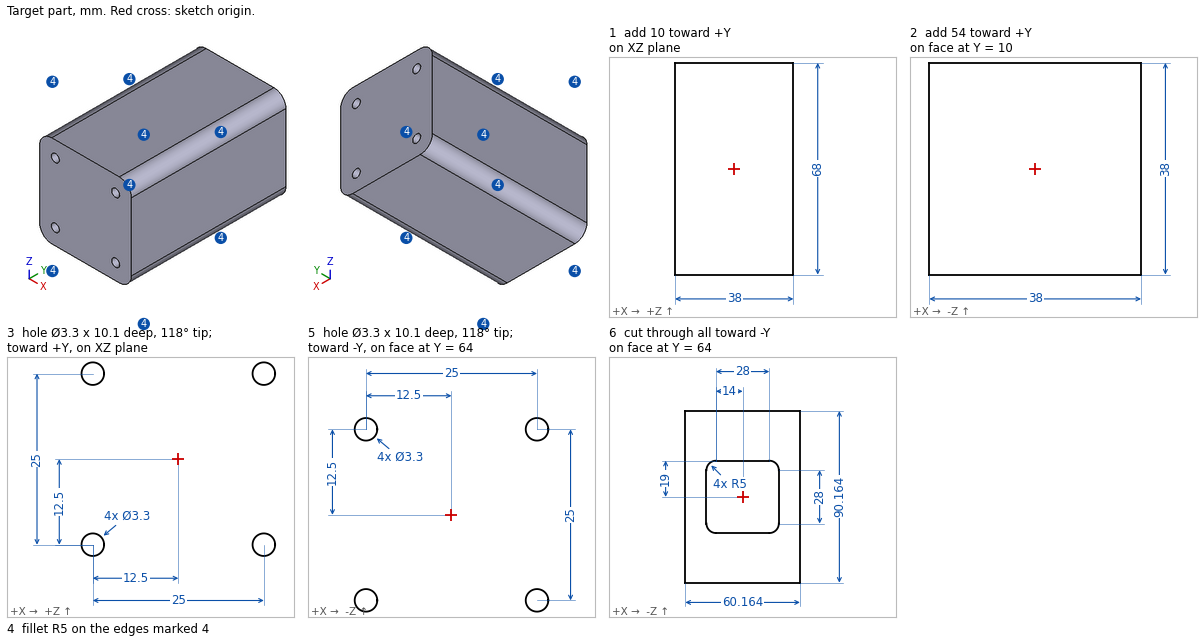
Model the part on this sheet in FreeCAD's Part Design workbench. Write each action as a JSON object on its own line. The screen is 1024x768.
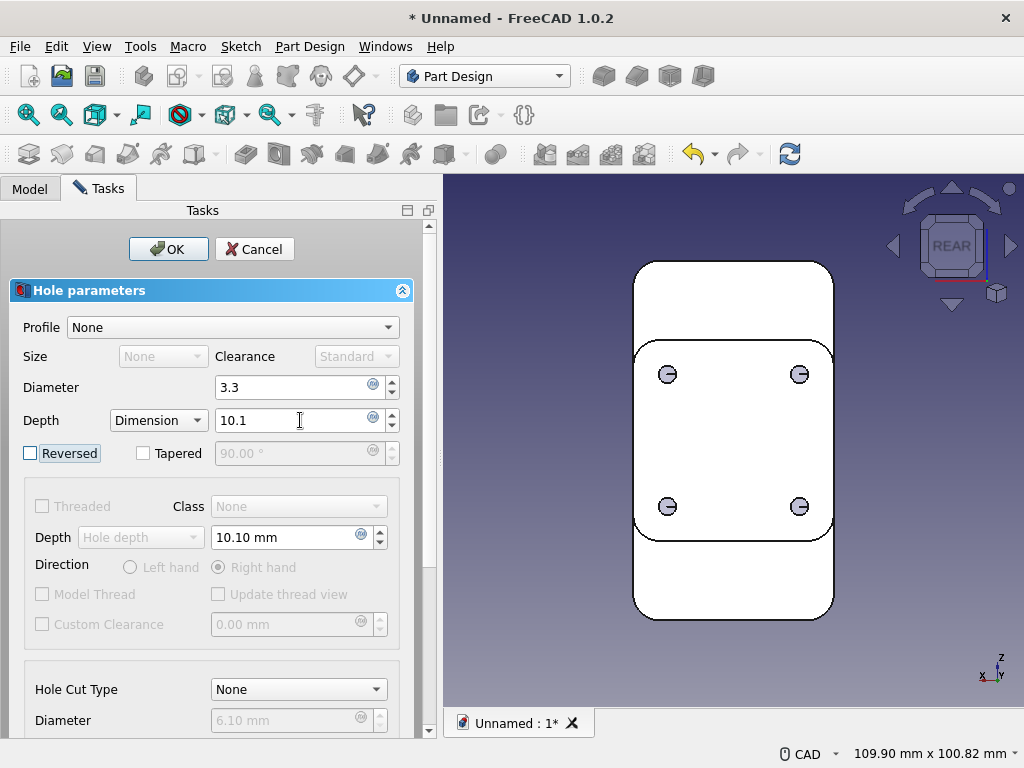
{"action": "left_click", "coordinate": [169, 249]}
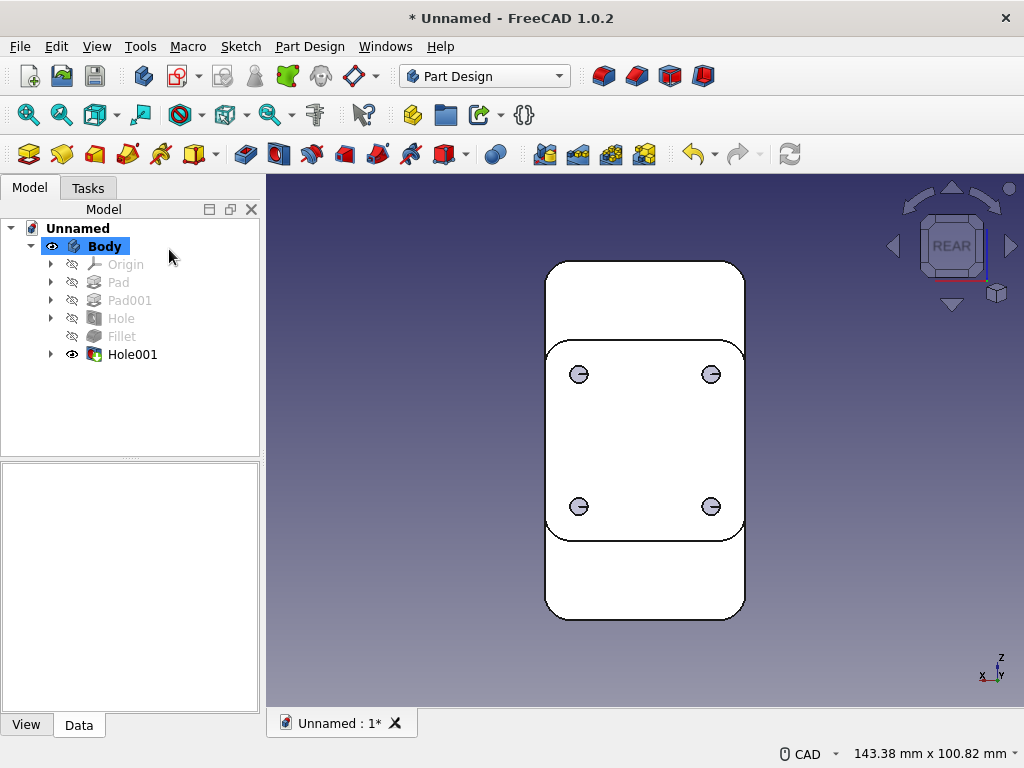
{"action": "left_click", "coordinate": [645, 440]}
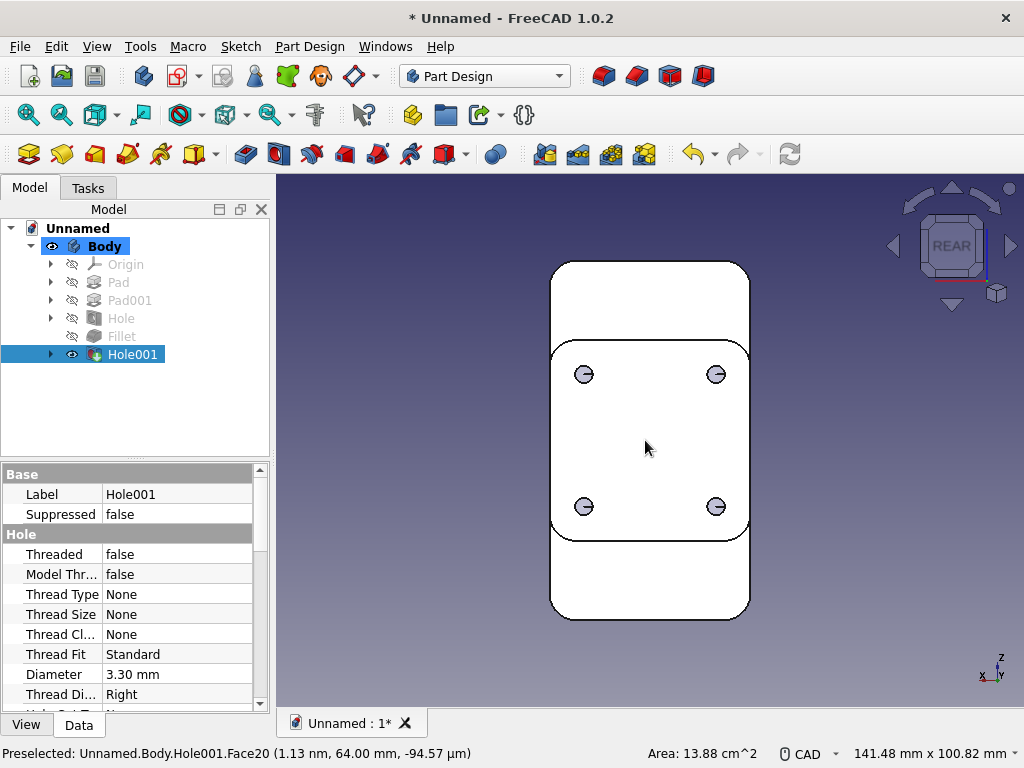
{"action": "left_click", "coordinate": [176, 76]}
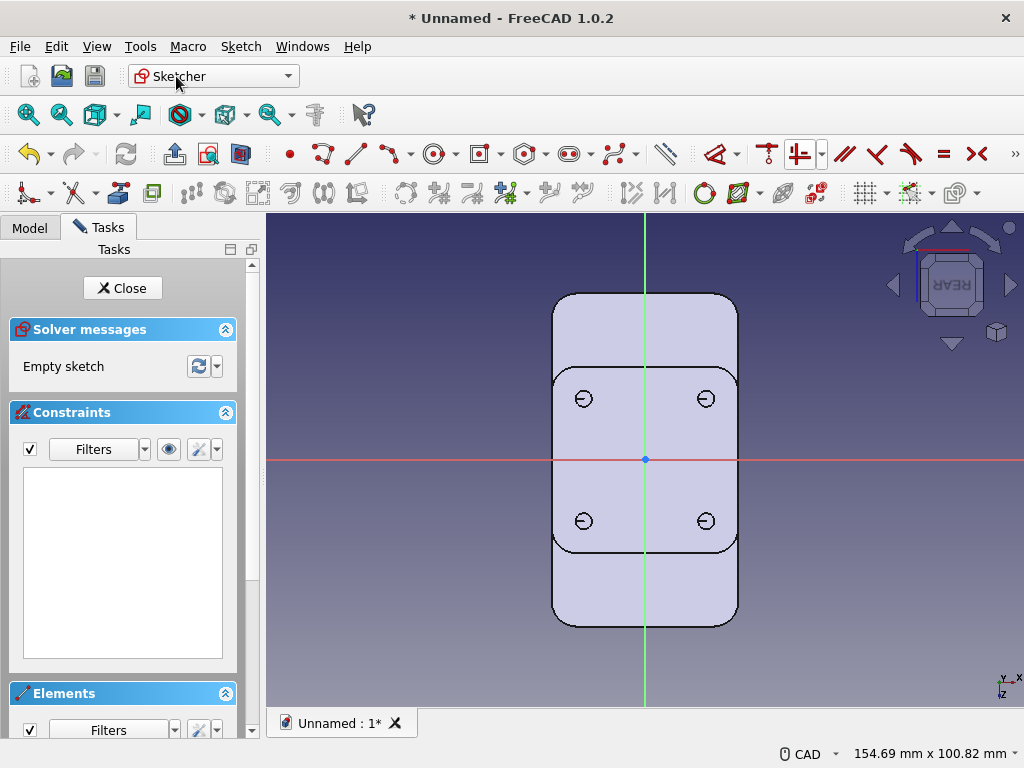
{"action": "scroll", "coordinate": [437, 460], "scroll_direction": "down", "scroll_amount": 2}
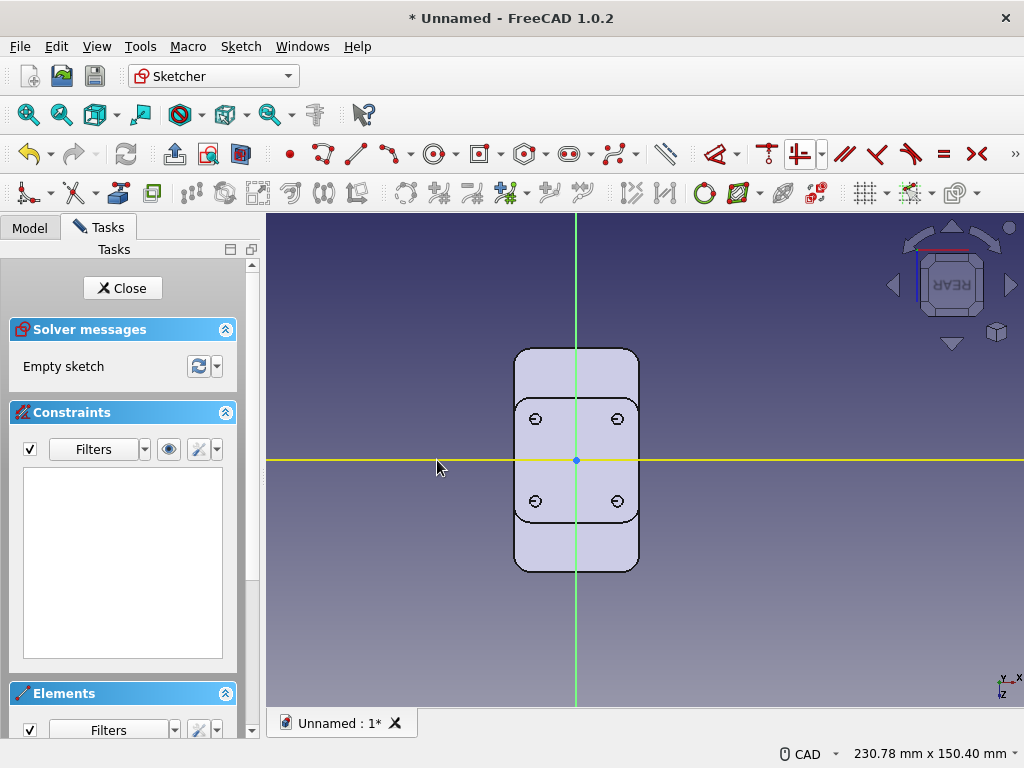
{"action": "key", "text": "g v"}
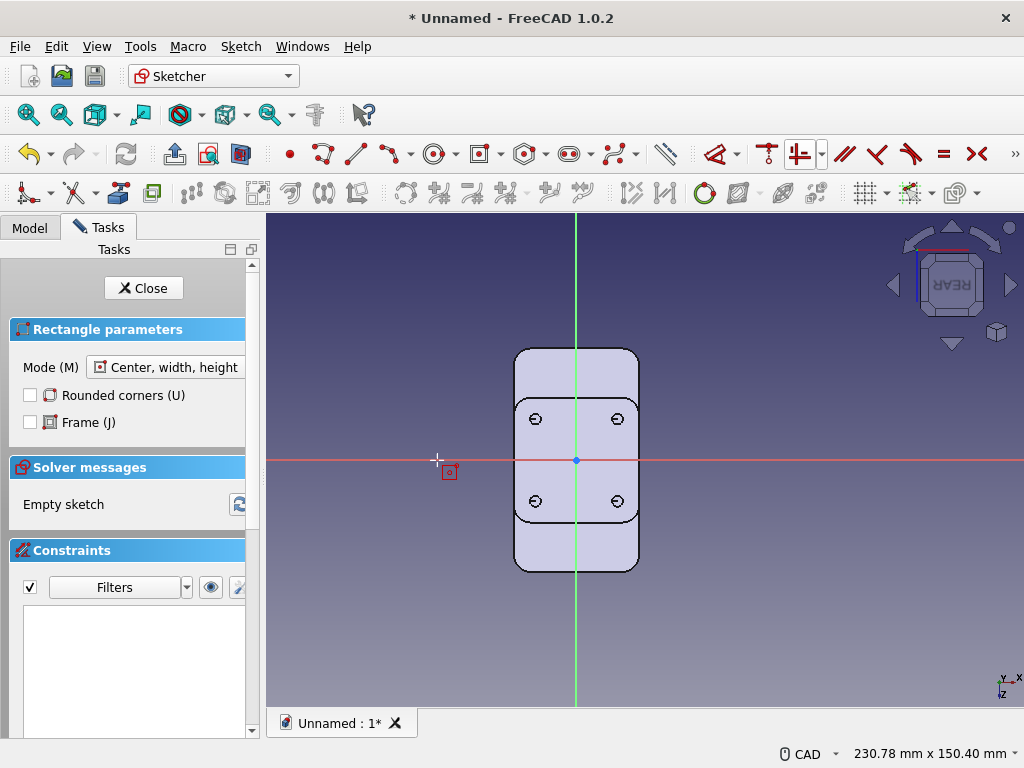
{"action": "left_click", "coordinate": [577, 460]}
{"action": "left_click", "coordinate": [675, 312]}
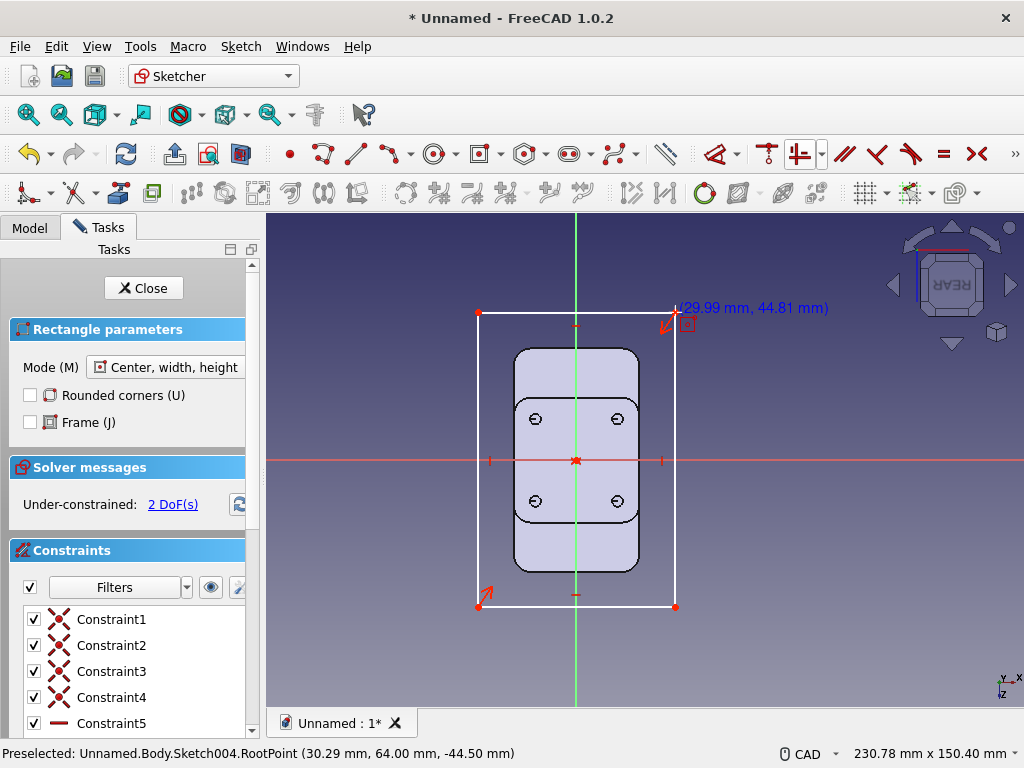
{"action": "left_click", "coordinate": [356, 154]}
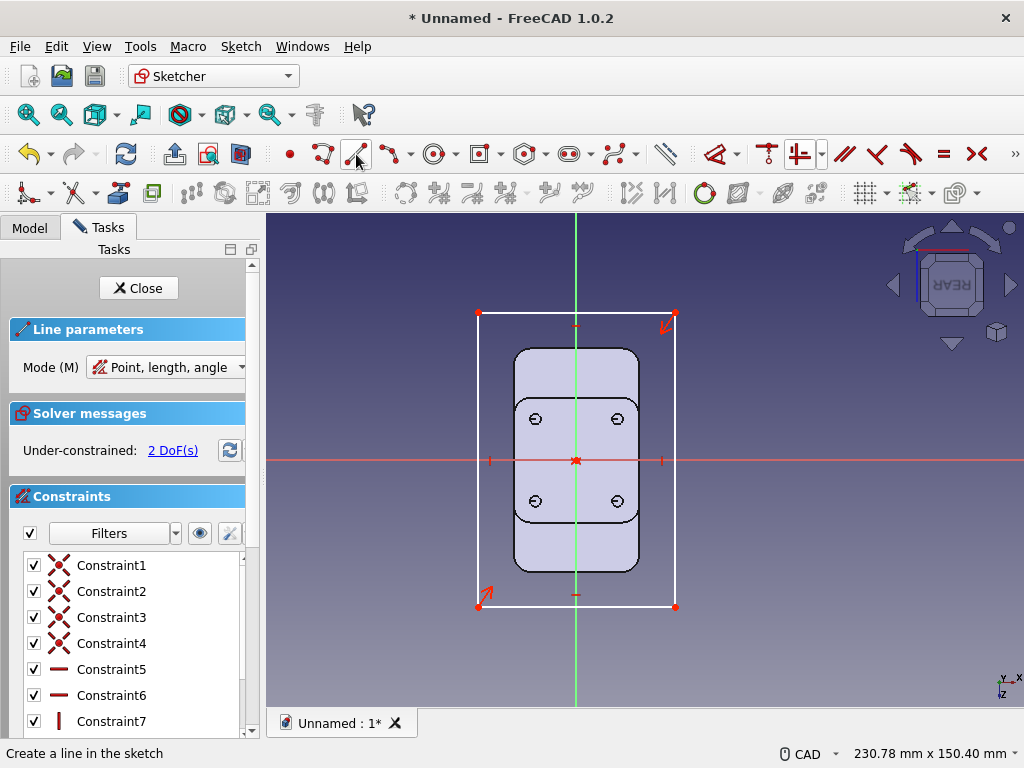
{"action": "left_click", "coordinate": [531, 398]}
{"action": "left_click", "coordinate": [622, 398]}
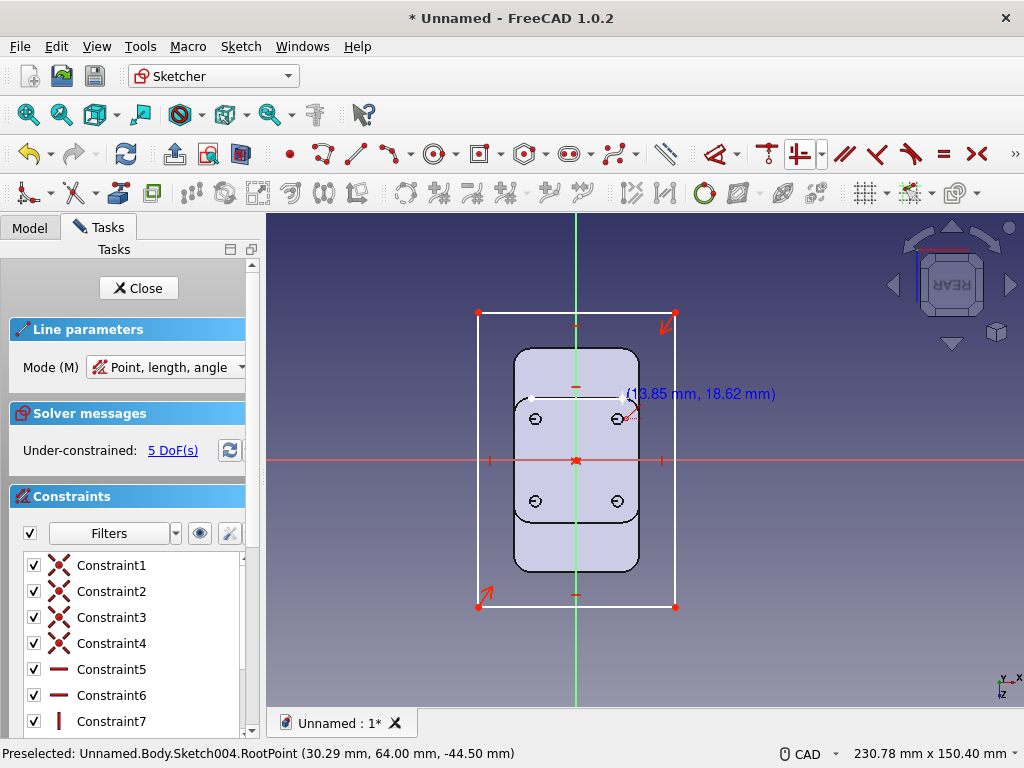
{"action": "left_click", "coordinate": [639, 414]}
{"action": "left_click", "coordinate": [639, 506]}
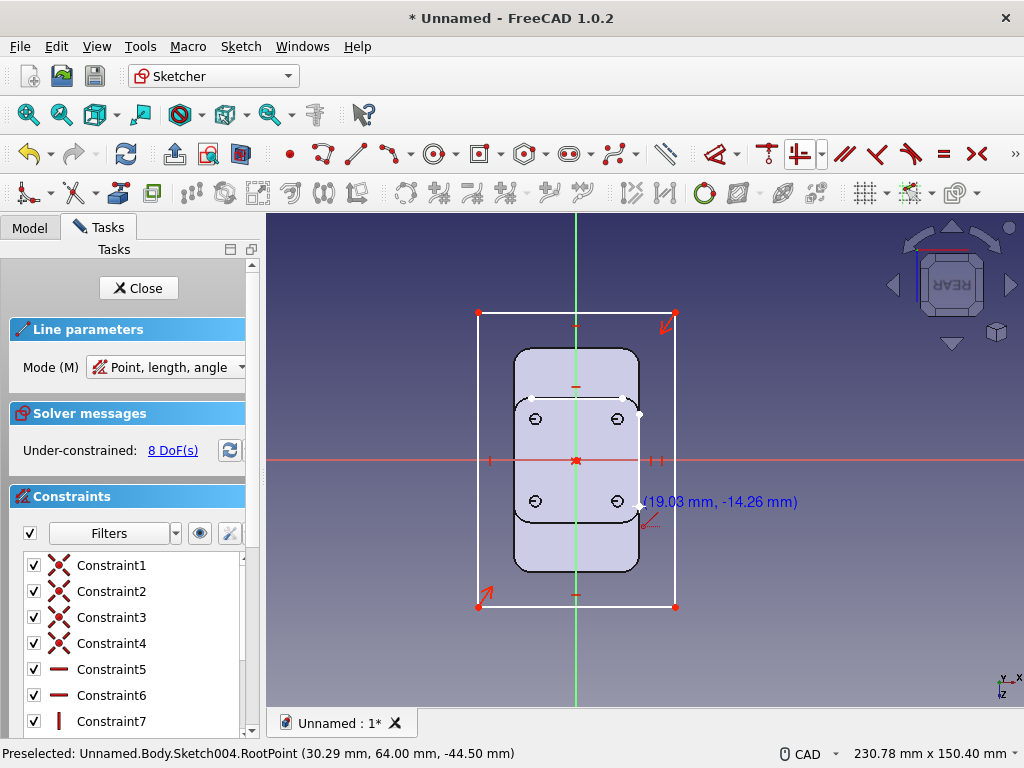
{"action": "left_click", "coordinate": [622, 523]}
{"action": "left_click", "coordinate": [531, 523]}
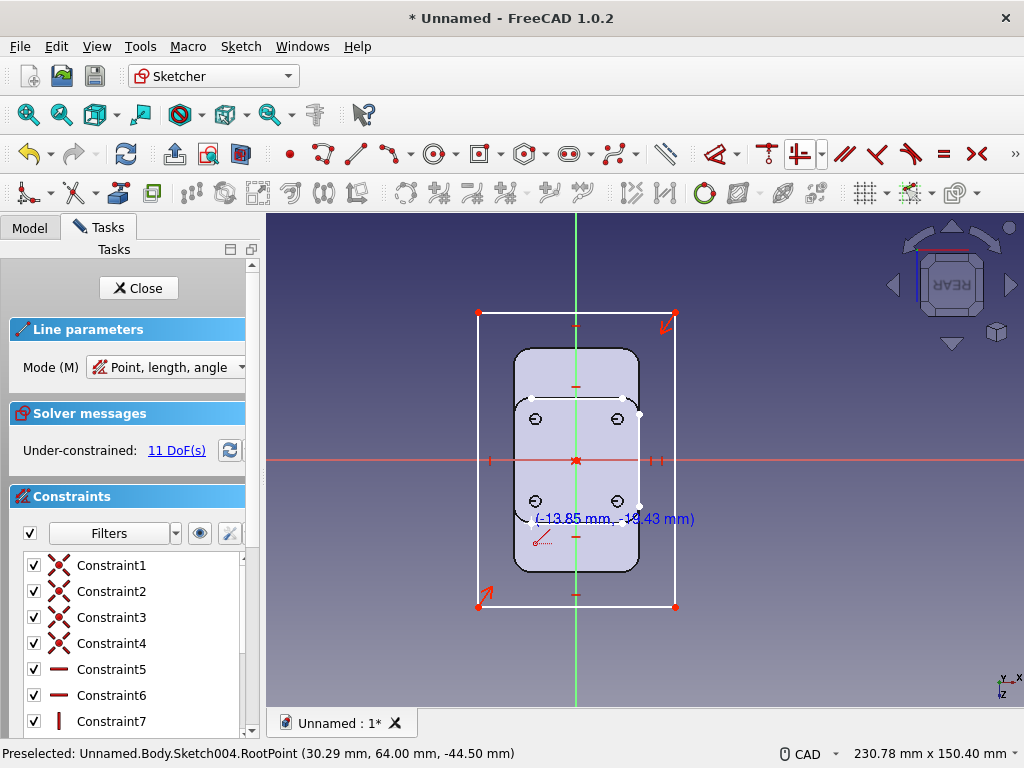
{"action": "left_click", "coordinate": [514, 506]}
{"action": "left_click", "coordinate": [514, 414]}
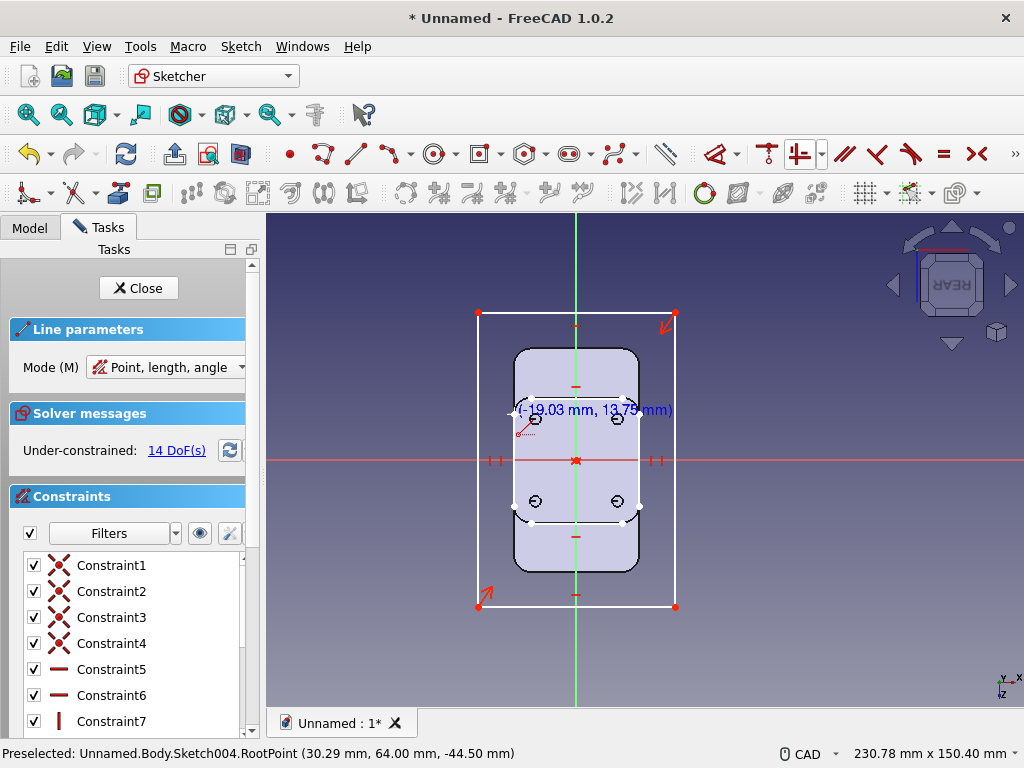
{"action": "key", "text": "g 3 a"}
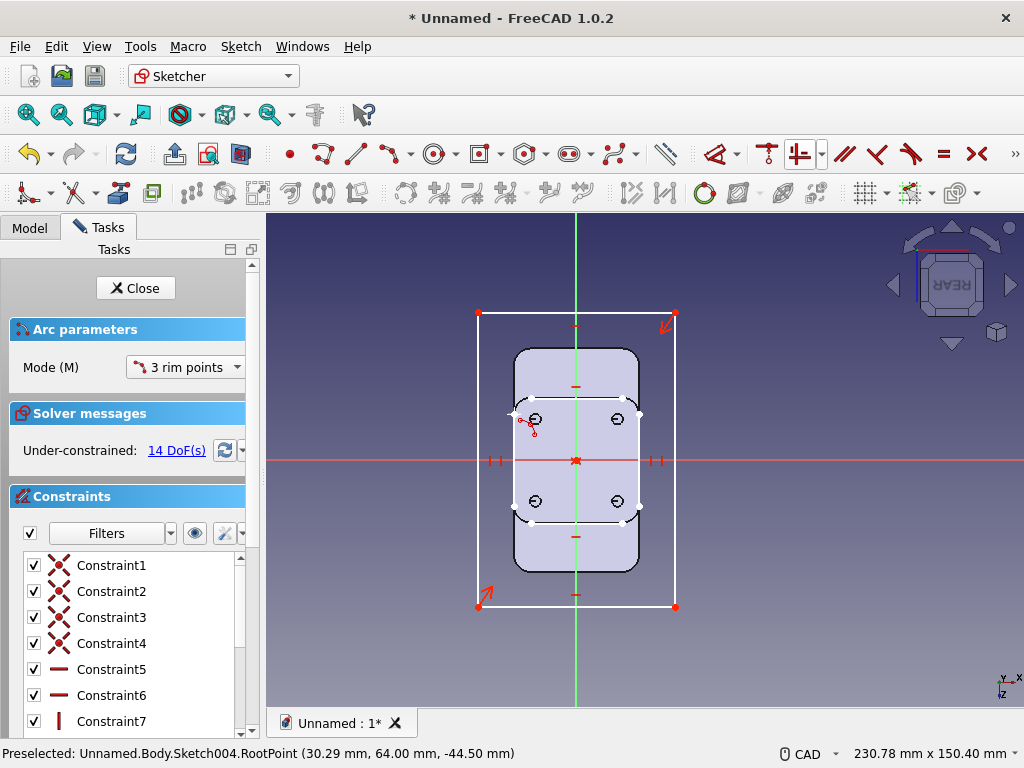
{"action": "left_click", "coordinate": [622, 399]}
{"action": "left_click", "coordinate": [639, 415]}